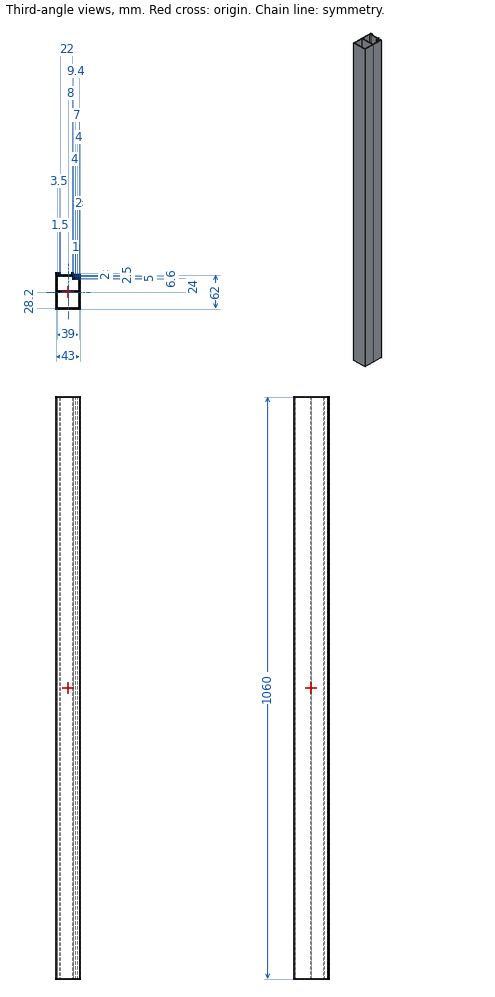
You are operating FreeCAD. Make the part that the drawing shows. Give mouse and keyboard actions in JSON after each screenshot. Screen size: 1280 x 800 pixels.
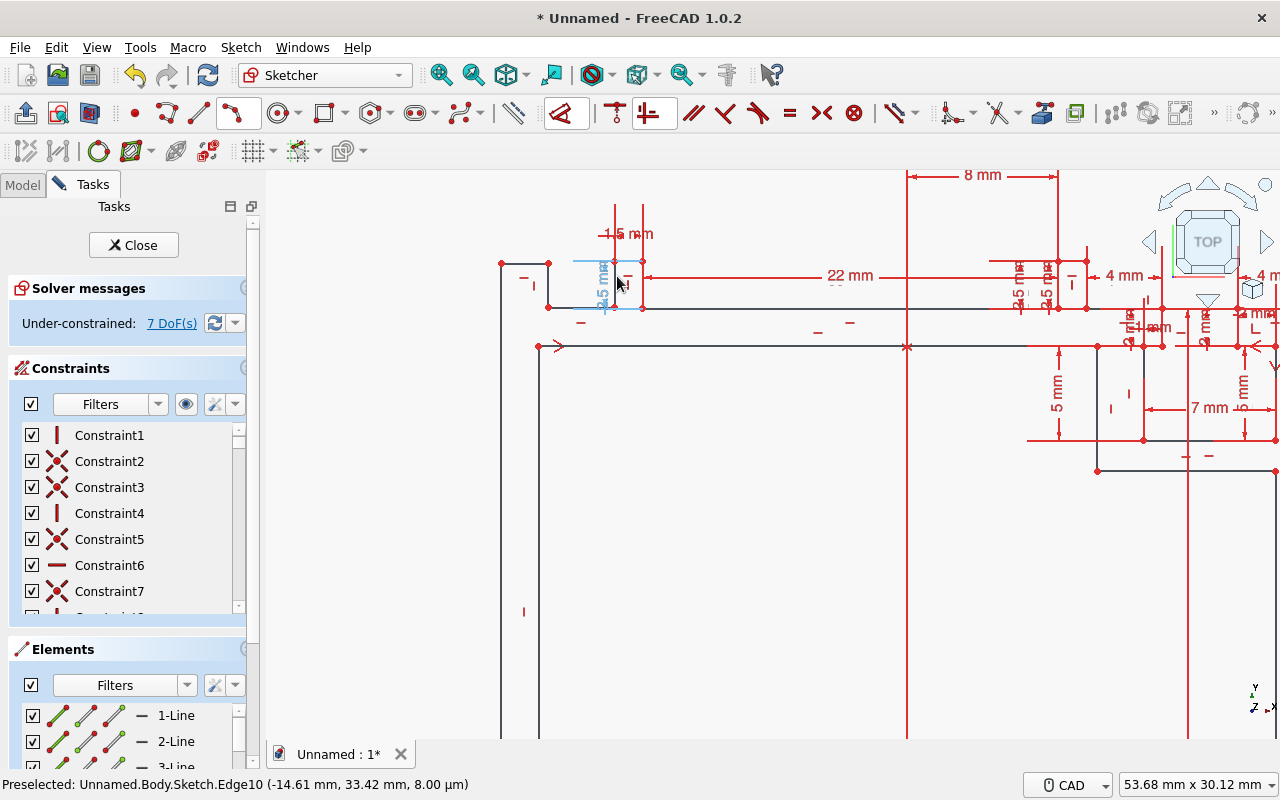
{"action": "left_click", "coordinate": [615, 275]}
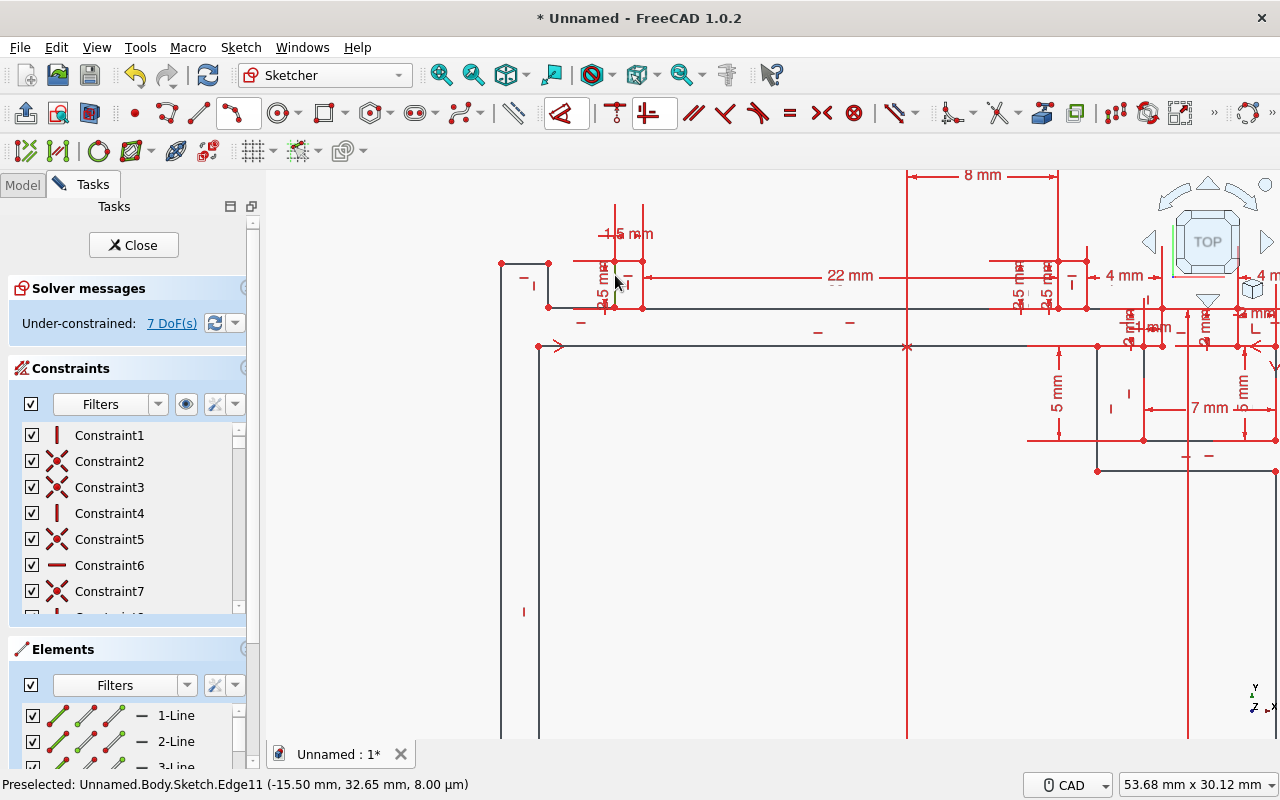
{"action": "left_click", "coordinate": [584, 114]}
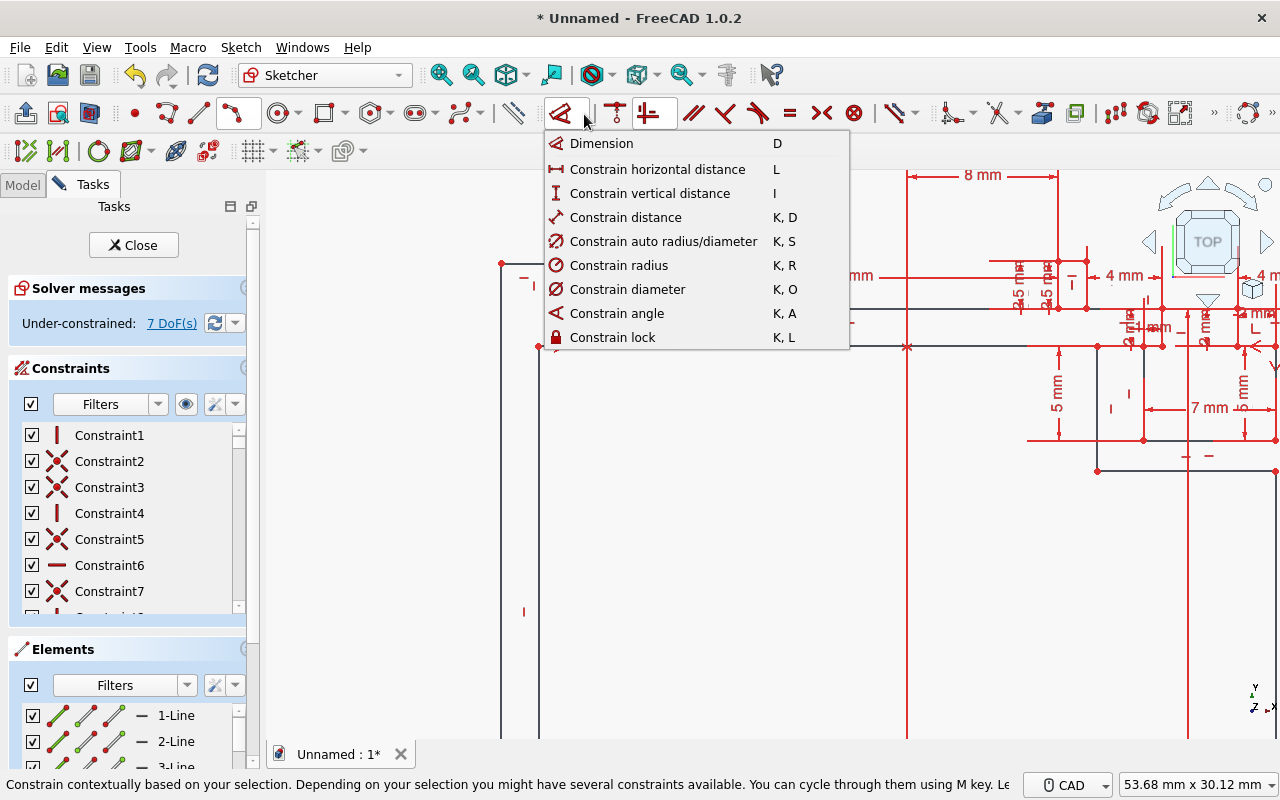
{"action": "left_click", "coordinate": [697, 193]}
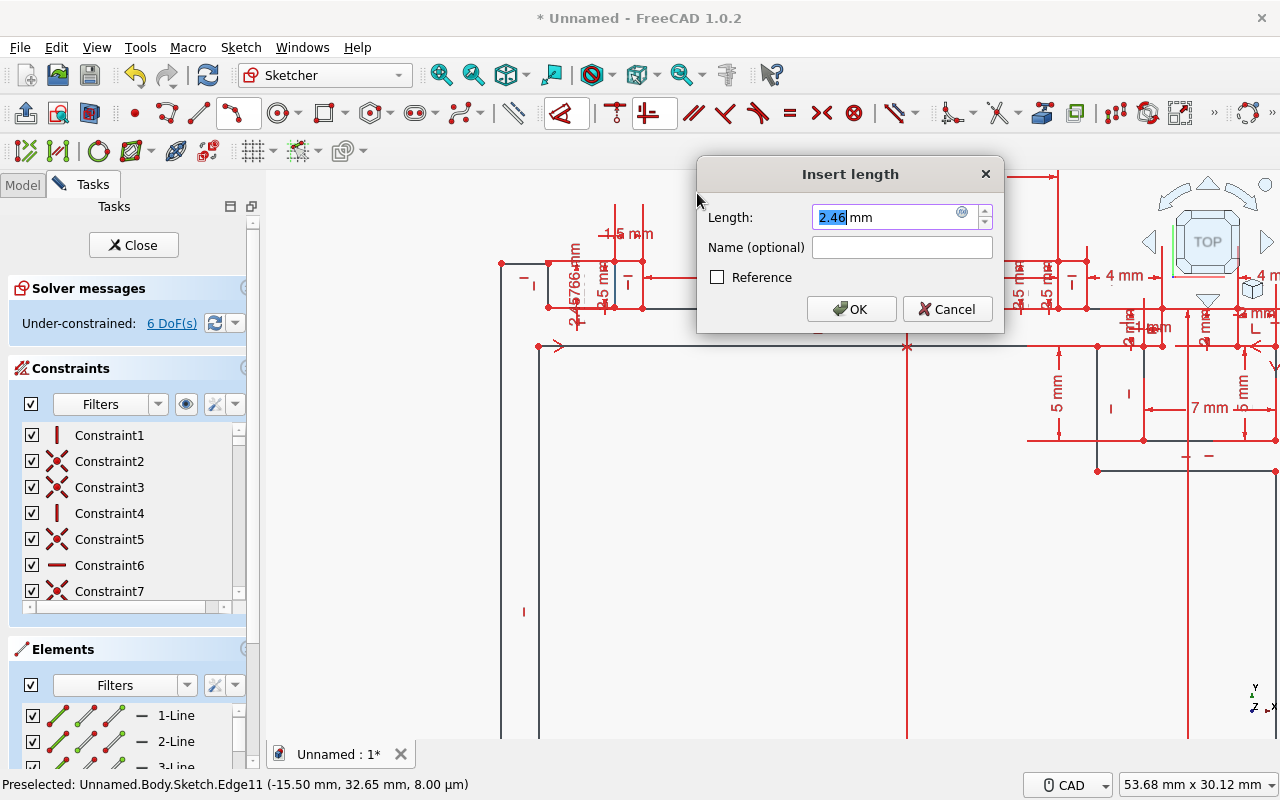
{"action": "type", "text": "2.5"}
{"action": "key", "text": "Return"}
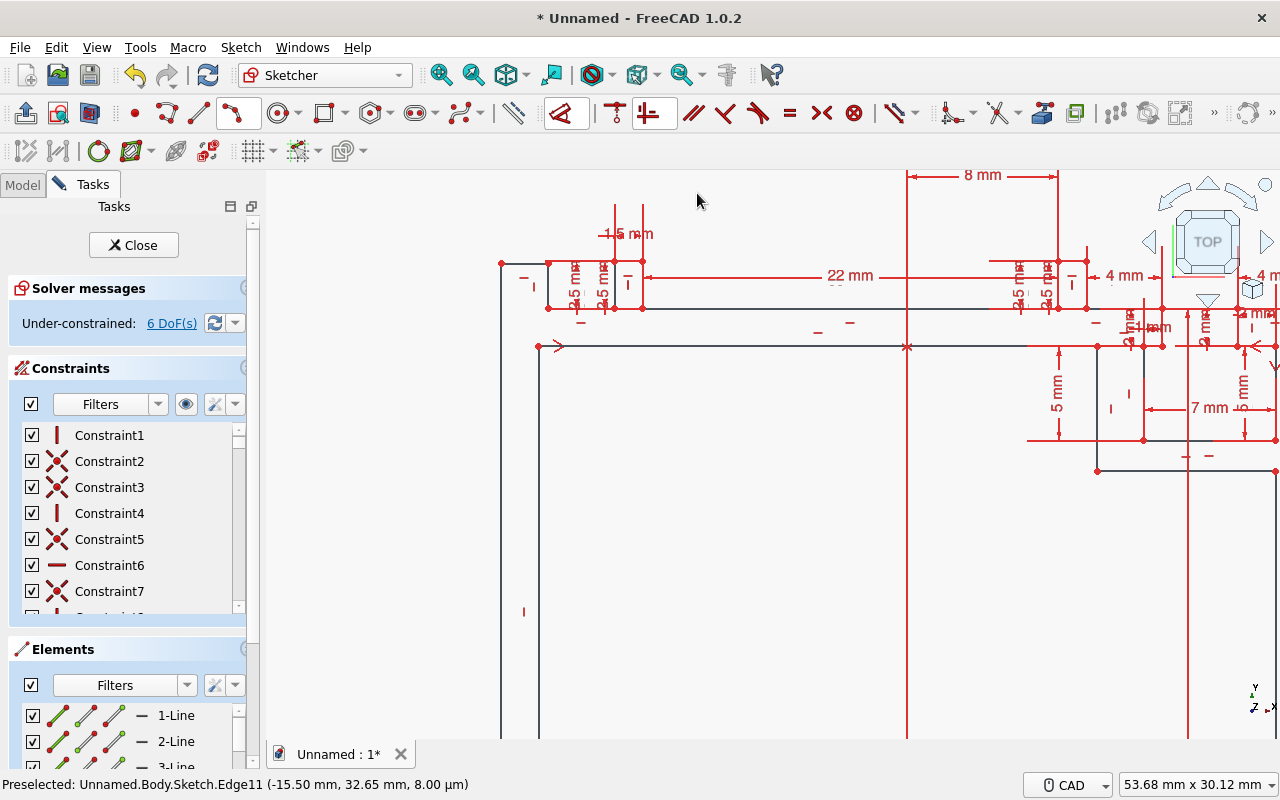
{"action": "left_click", "coordinate": [595, 309]}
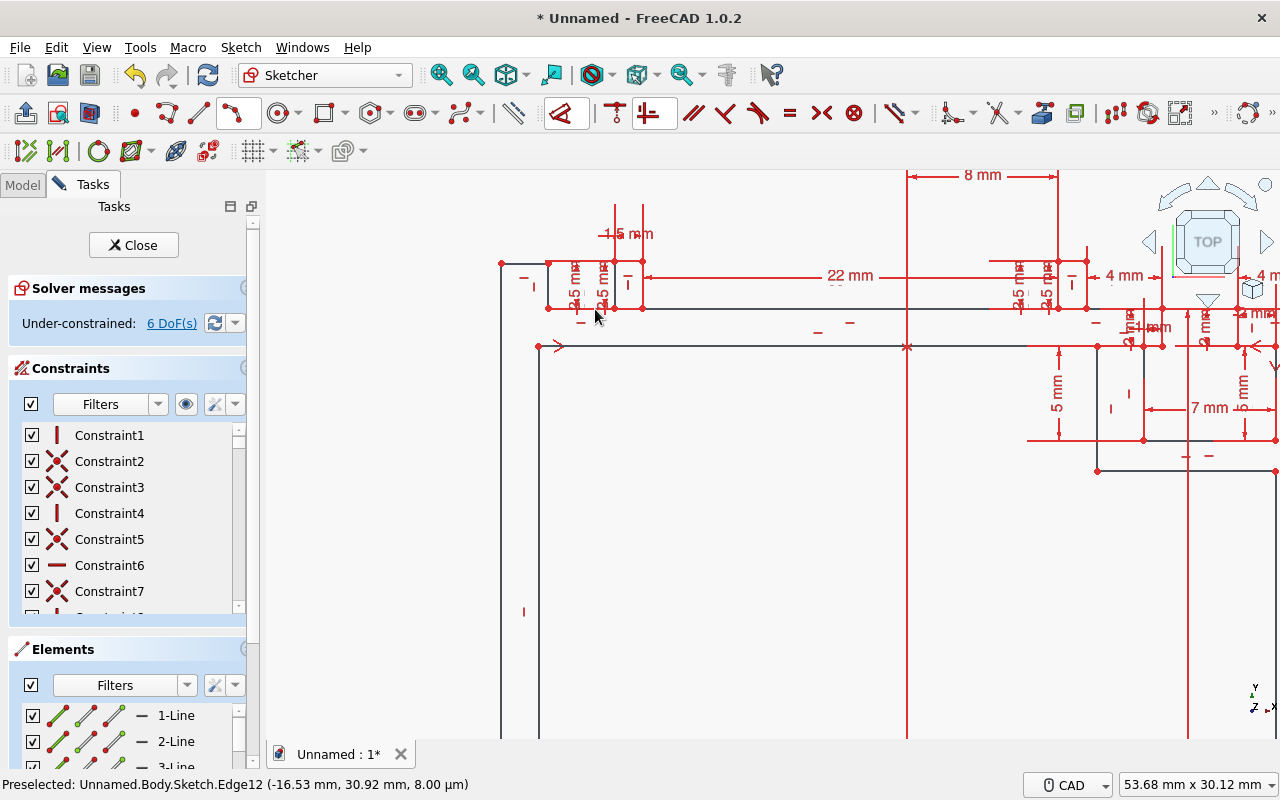
{"action": "key", "text": "l"}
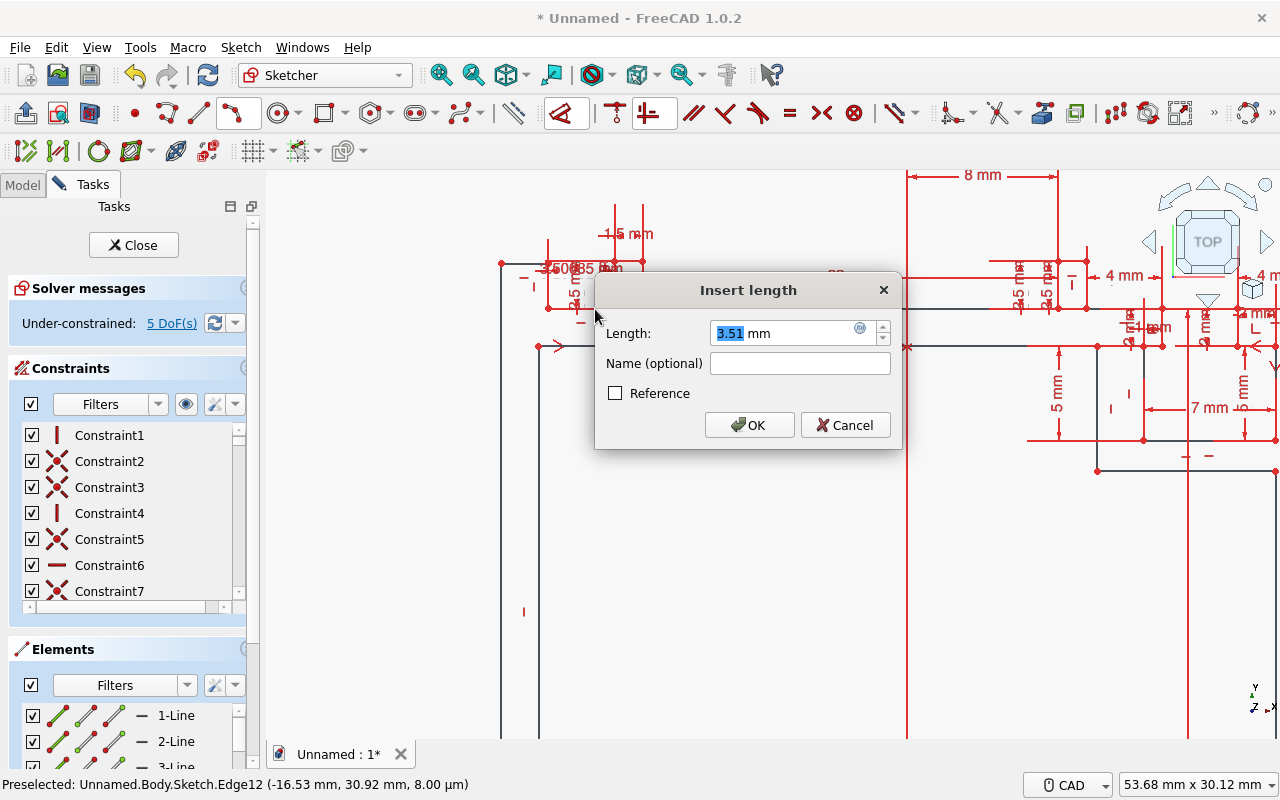
{"action": "type", "text": "3.5"}
{"action": "key", "text": "Return"}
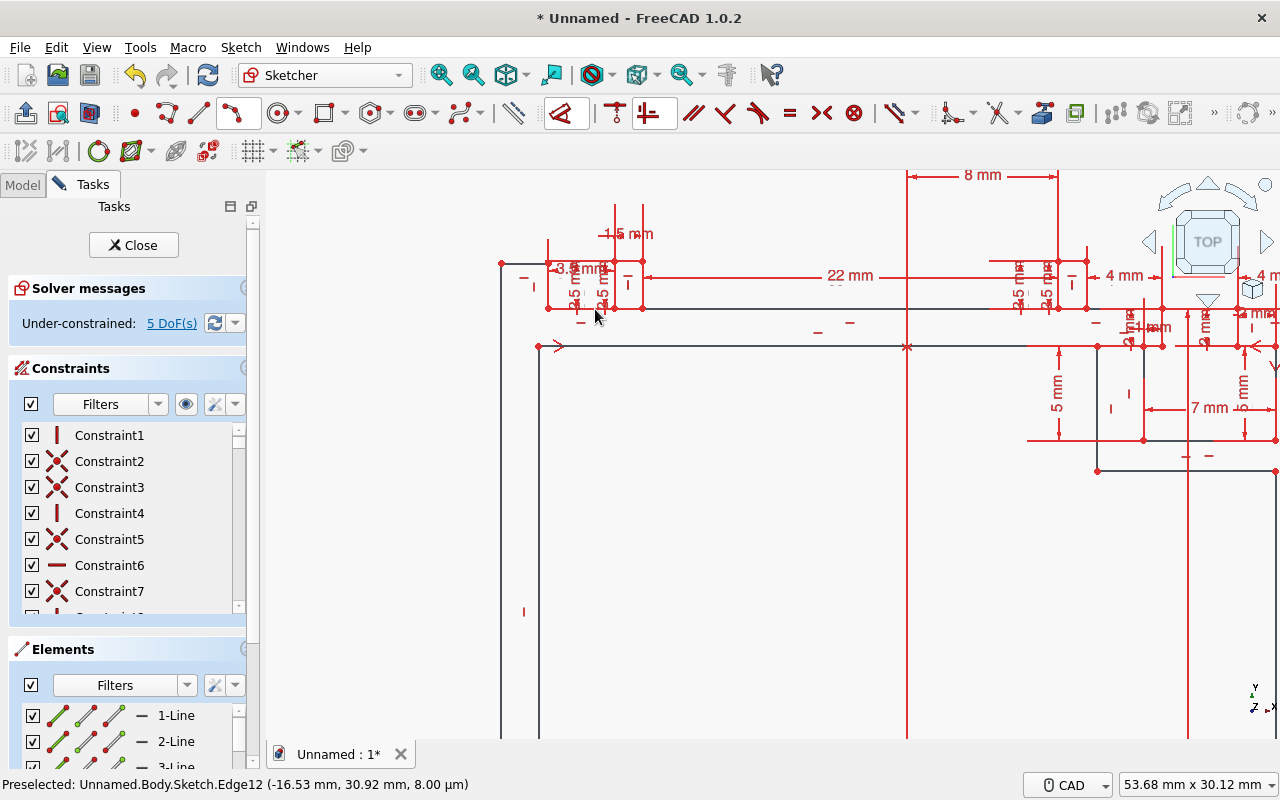
{"action": "left_click", "coordinate": [548, 295]}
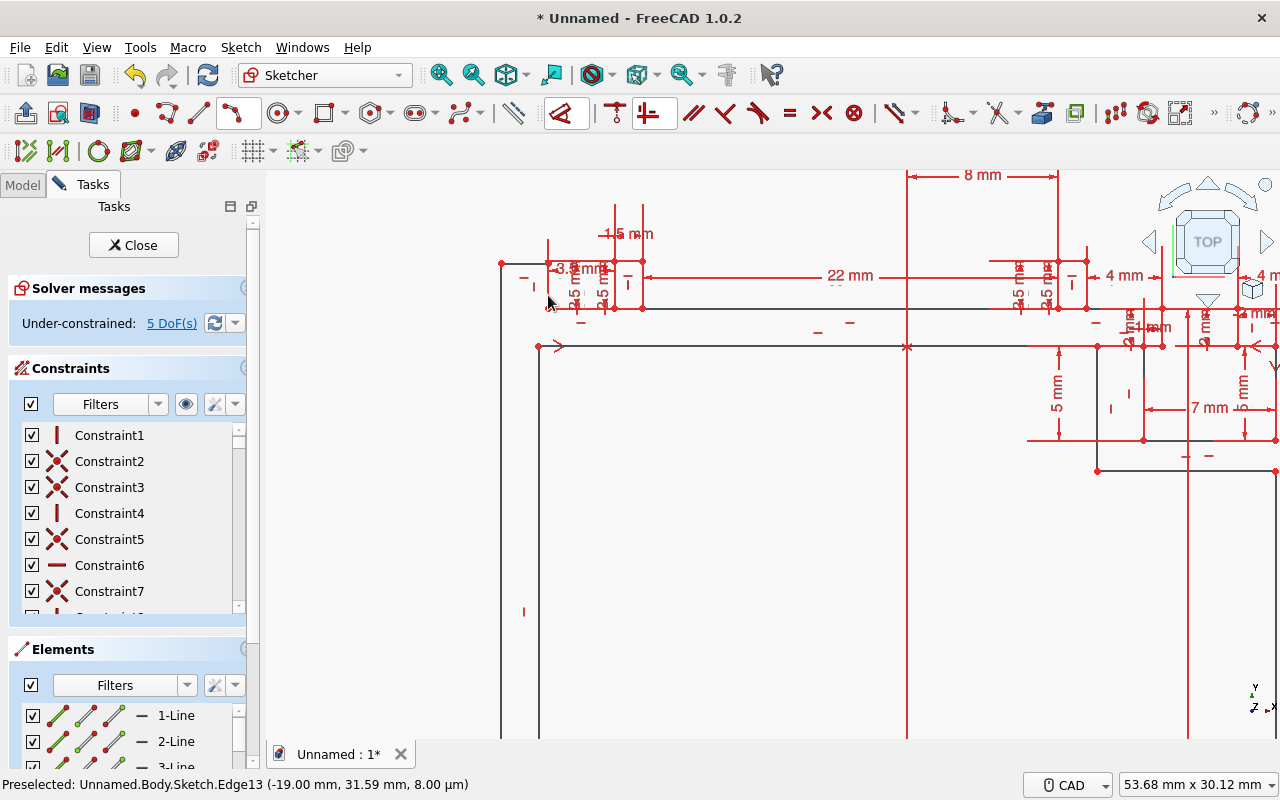
{"action": "key", "text": "i"}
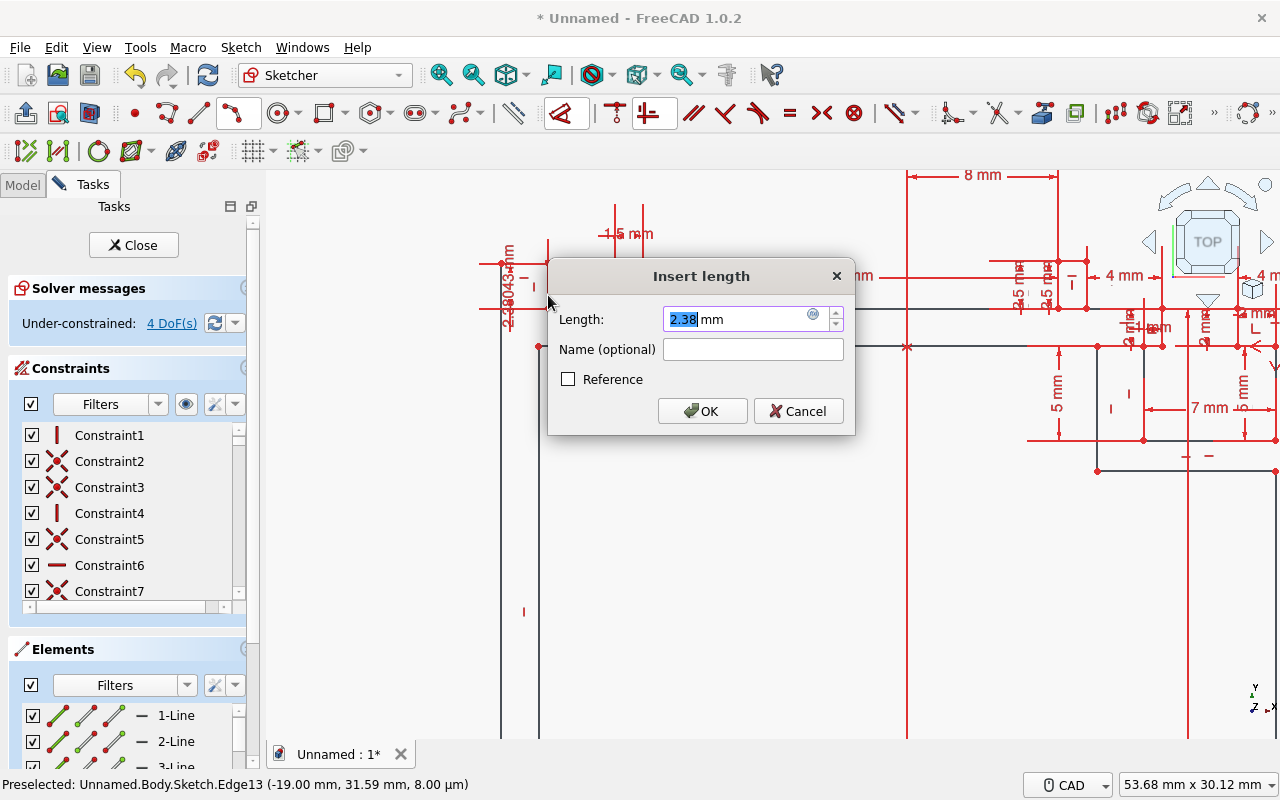
{"action": "type", "text": "2.5"}
{"action": "key", "text": "Return"}